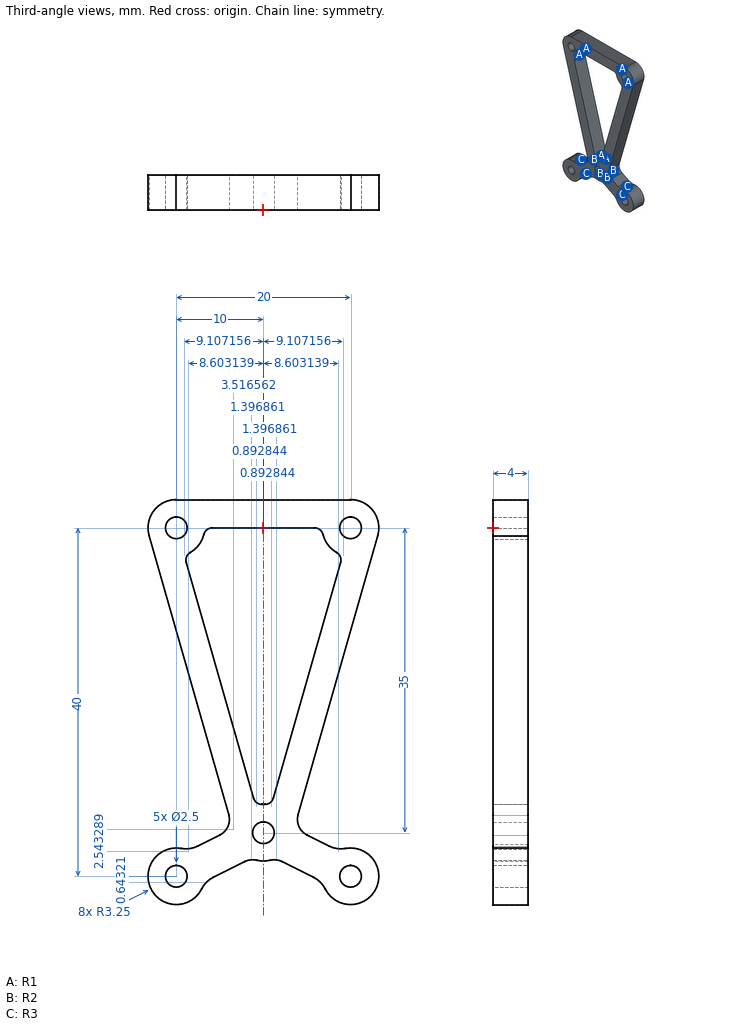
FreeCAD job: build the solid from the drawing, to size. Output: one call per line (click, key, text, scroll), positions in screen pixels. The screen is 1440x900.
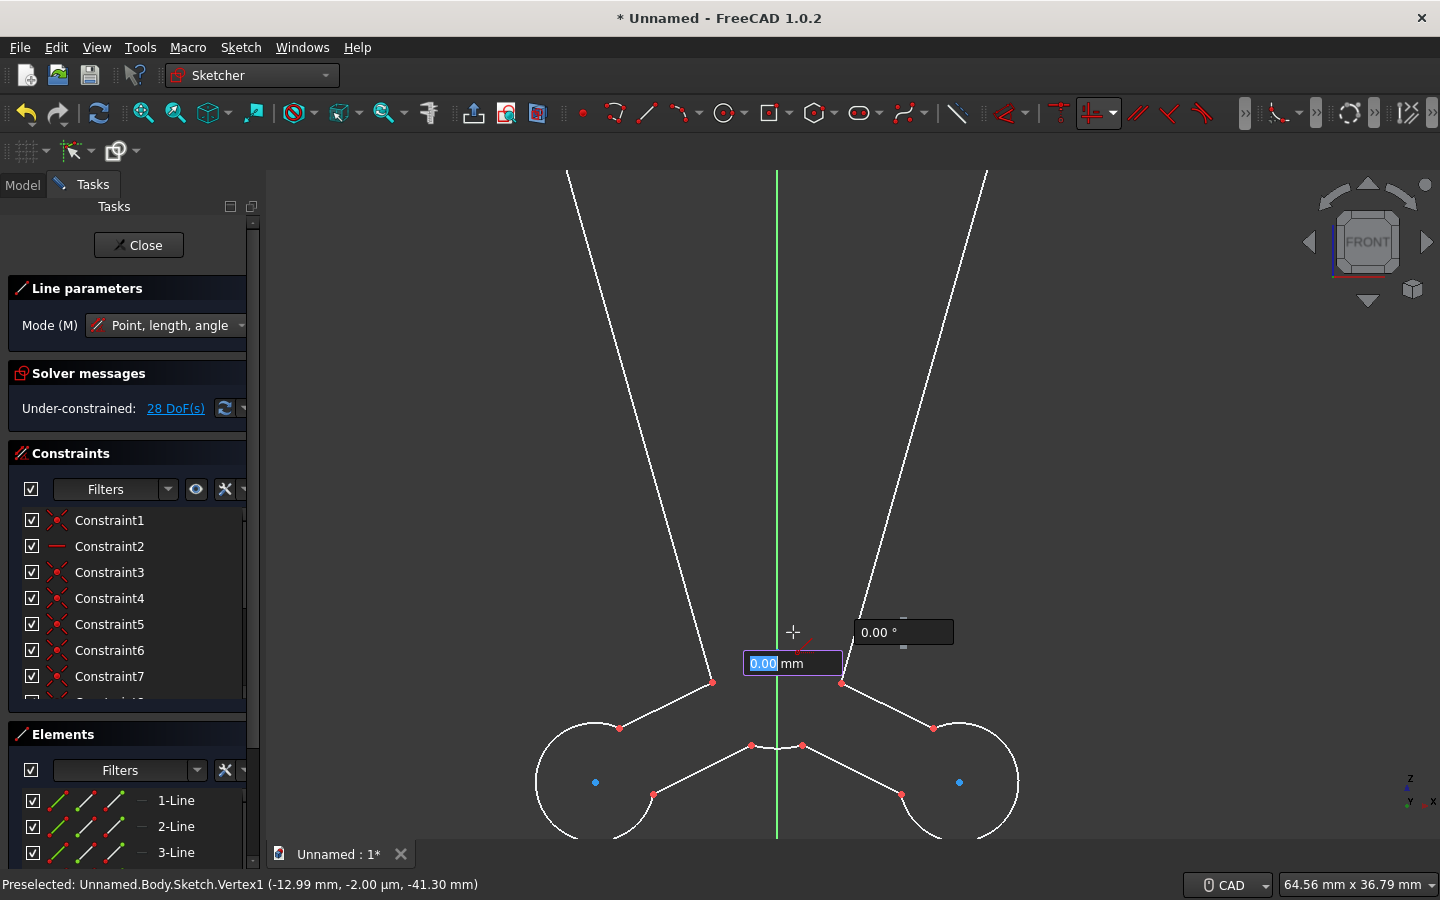
scroll(794, 632, down, 3)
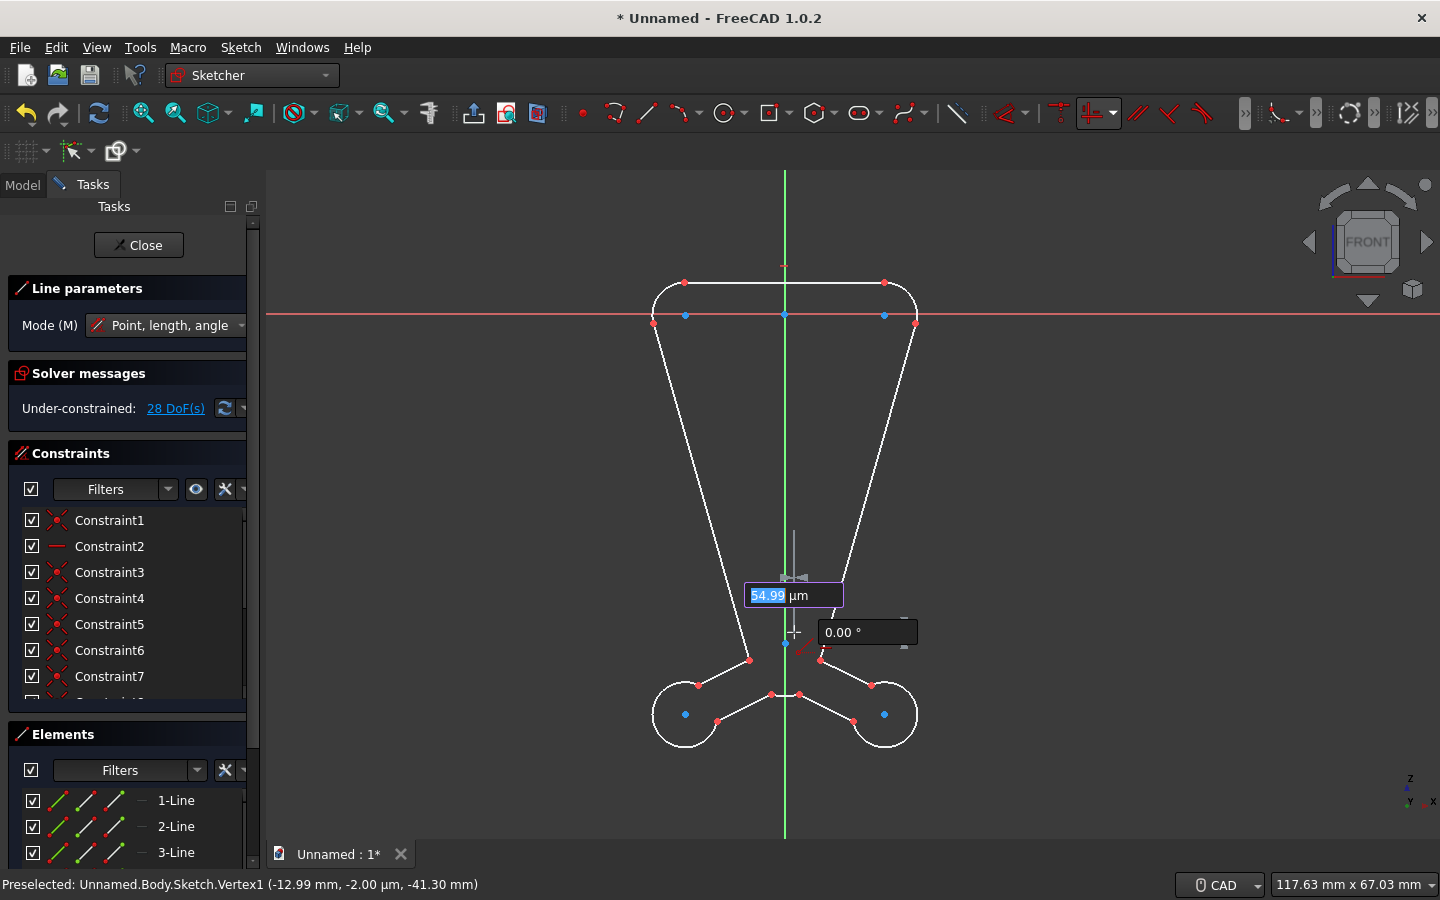
click(876, 346)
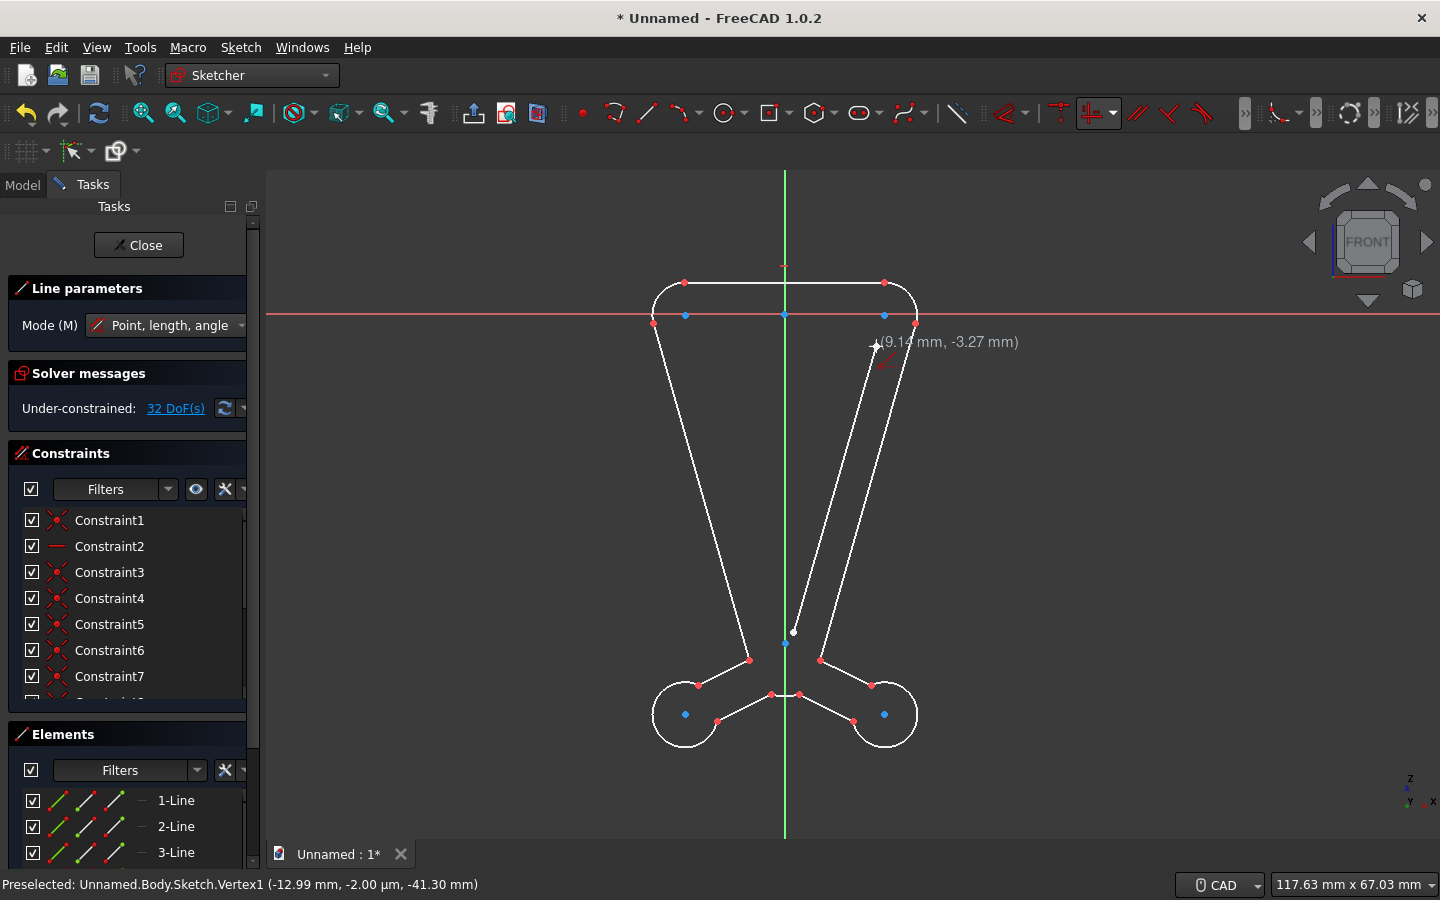
click(852, 314)
click(717, 323)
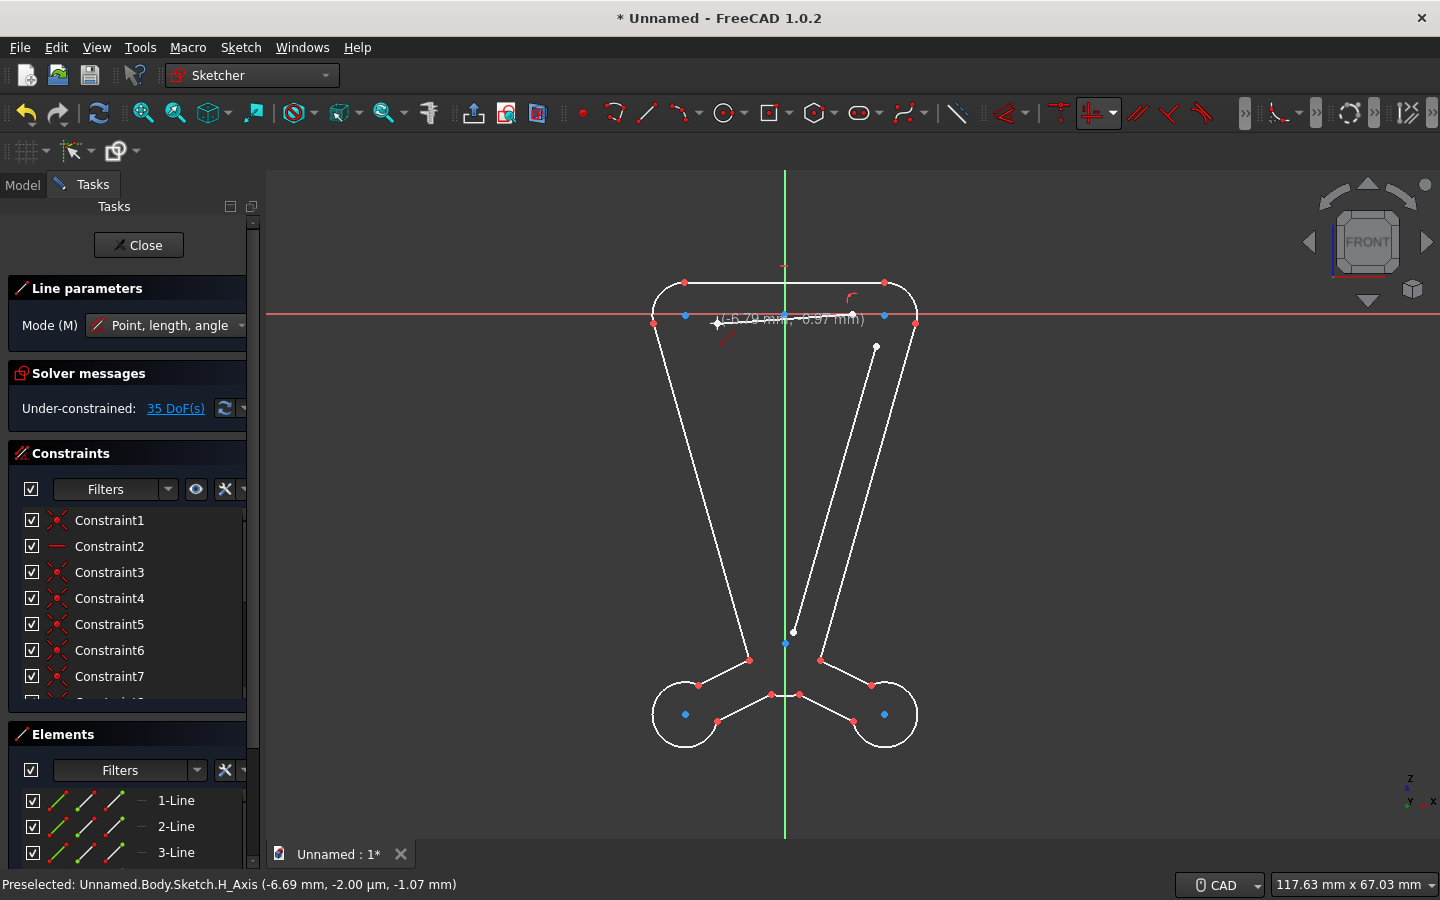
click(694, 346)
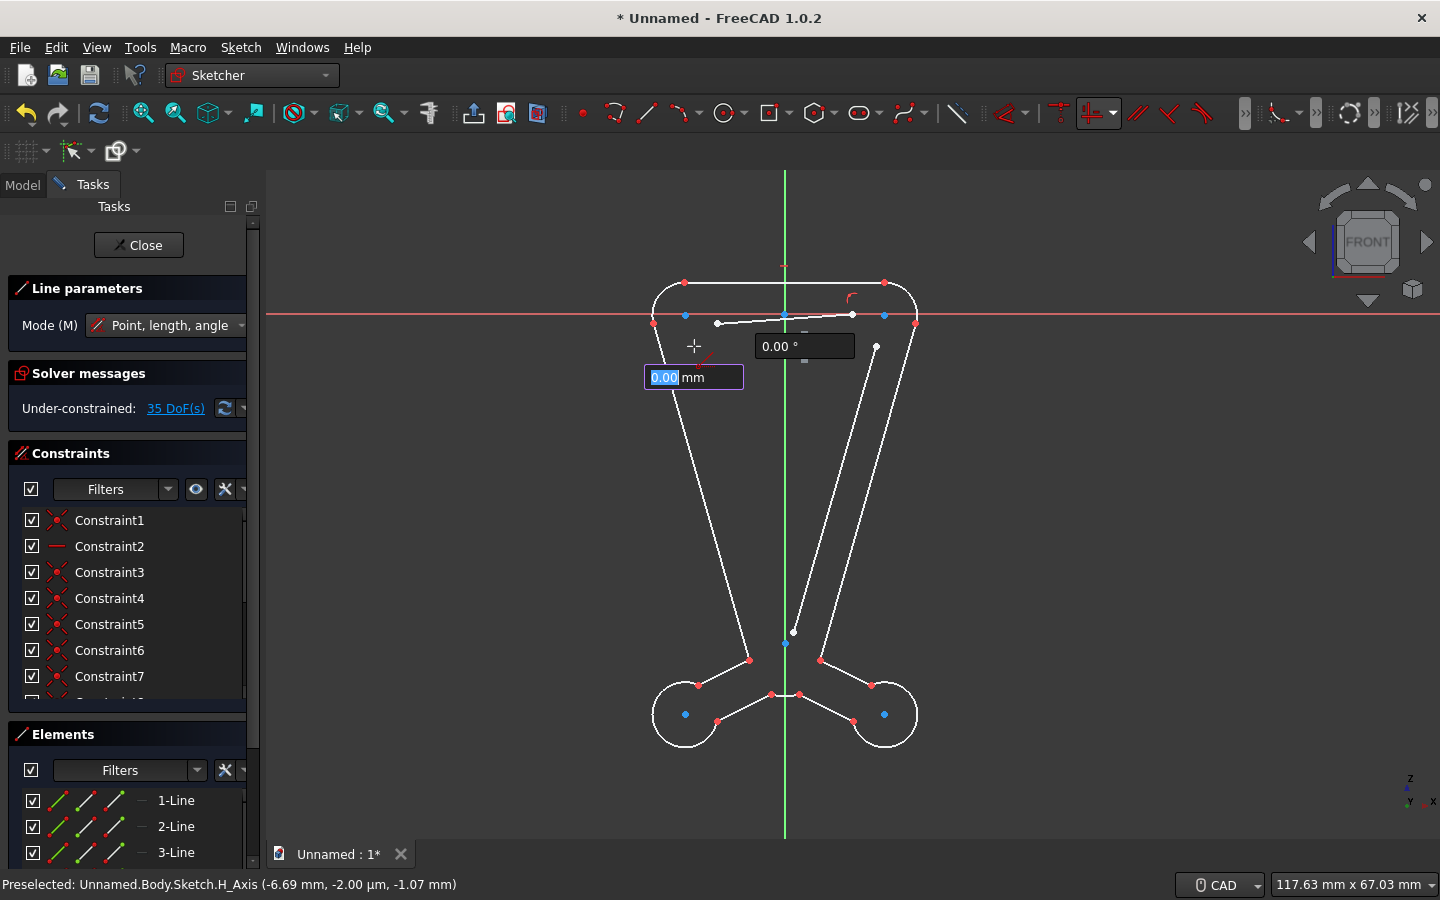
scroll(776, 632, up, 3)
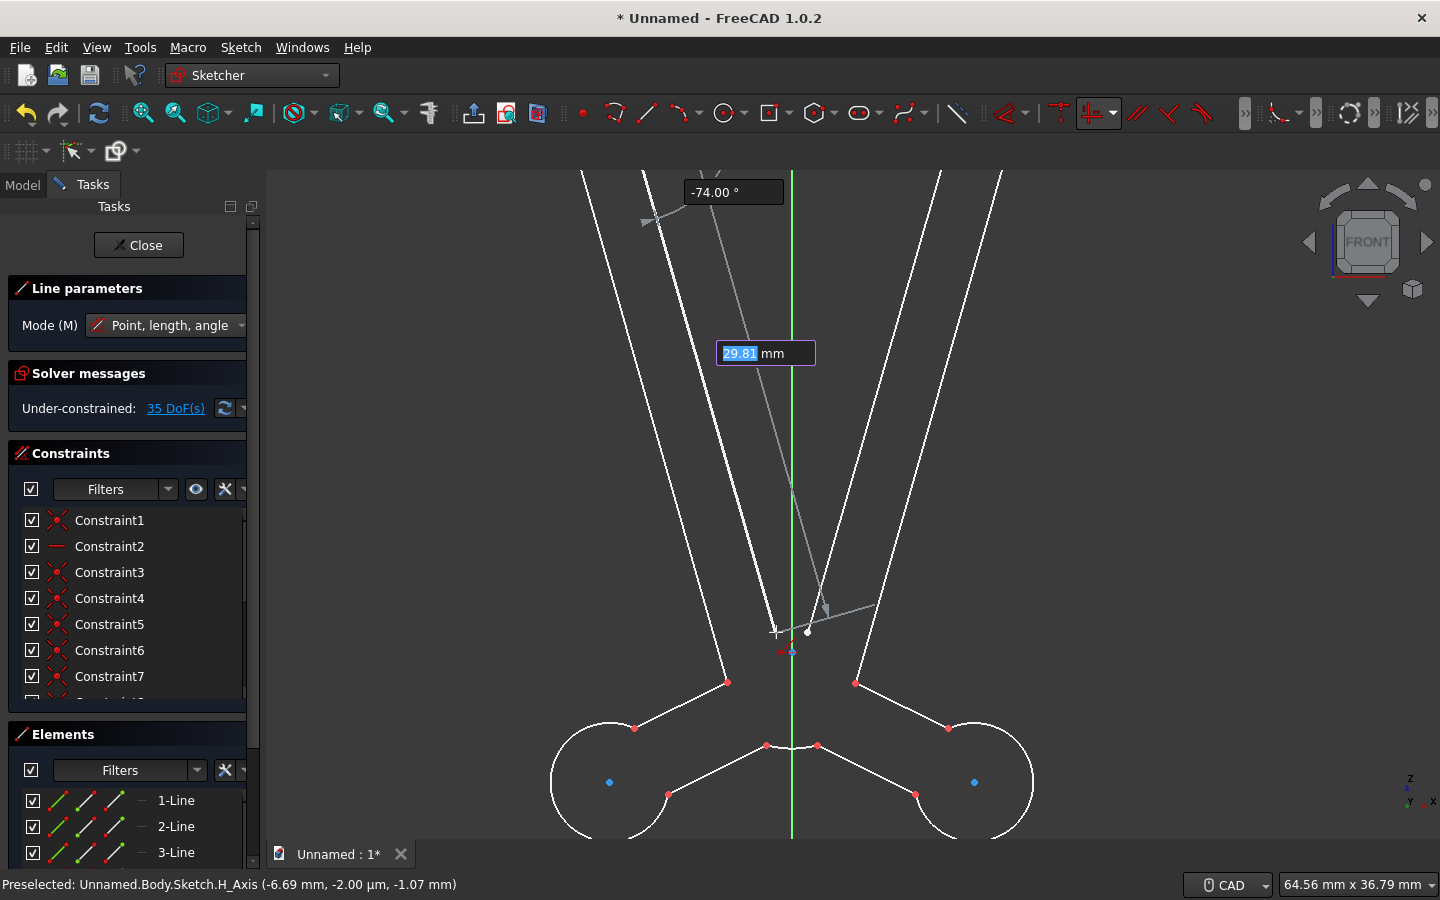
click(775, 632)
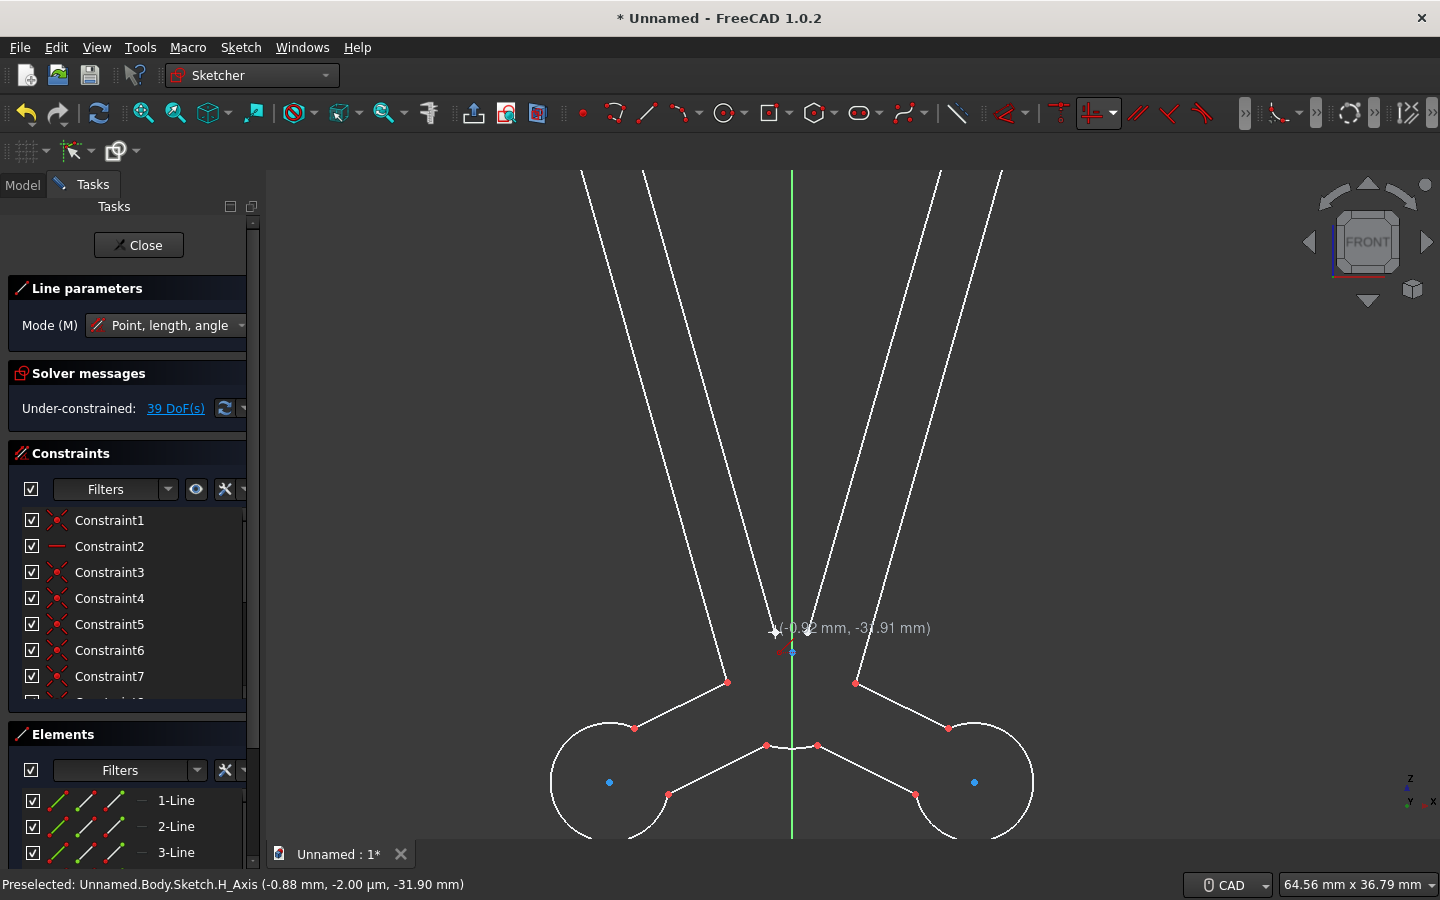
click(680, 114)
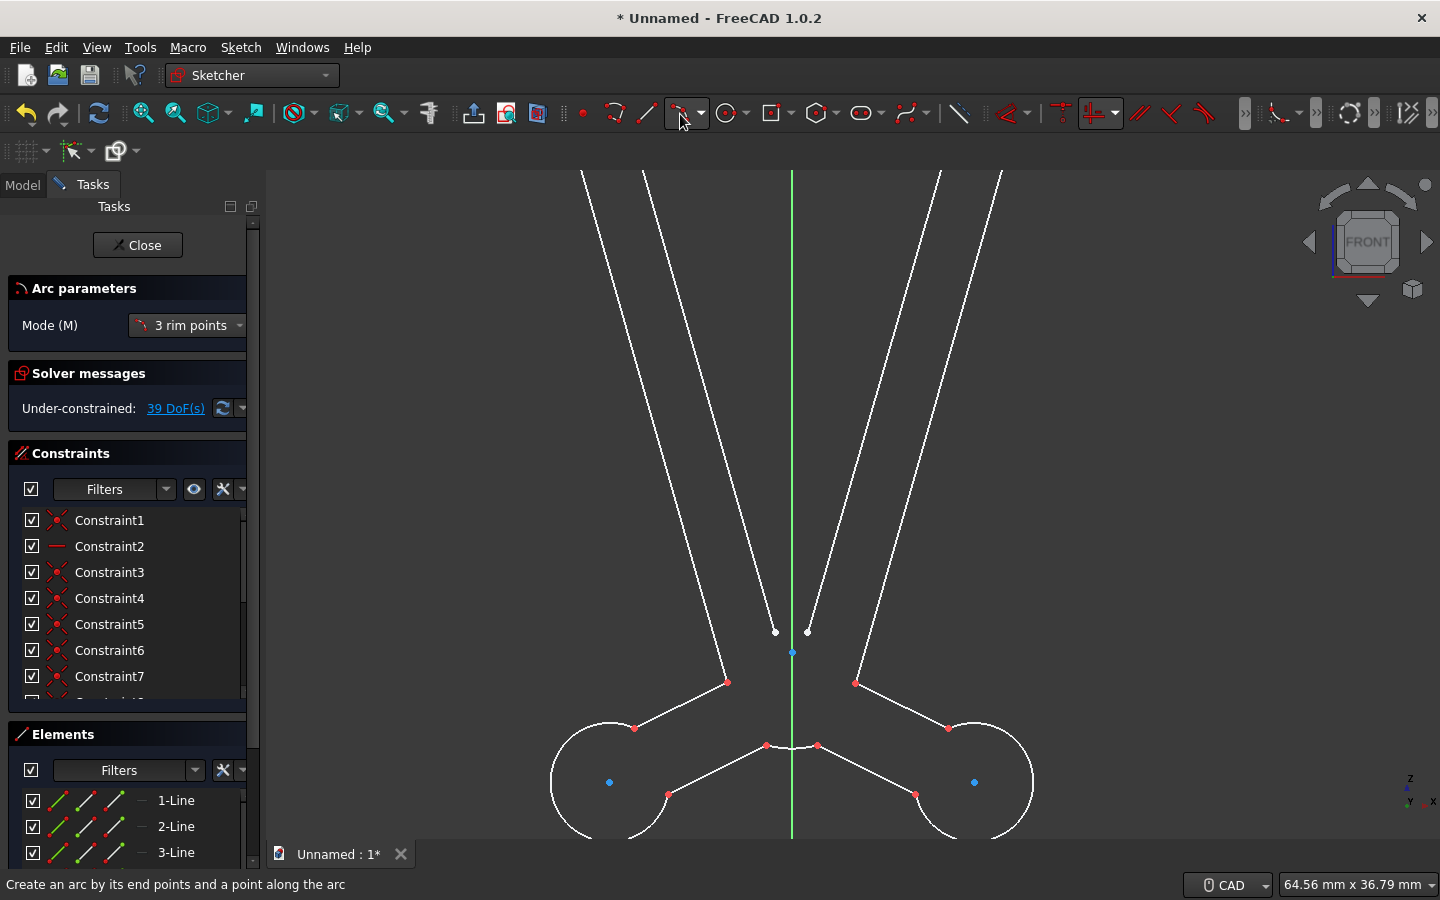
scroll(776, 632, down, 3)